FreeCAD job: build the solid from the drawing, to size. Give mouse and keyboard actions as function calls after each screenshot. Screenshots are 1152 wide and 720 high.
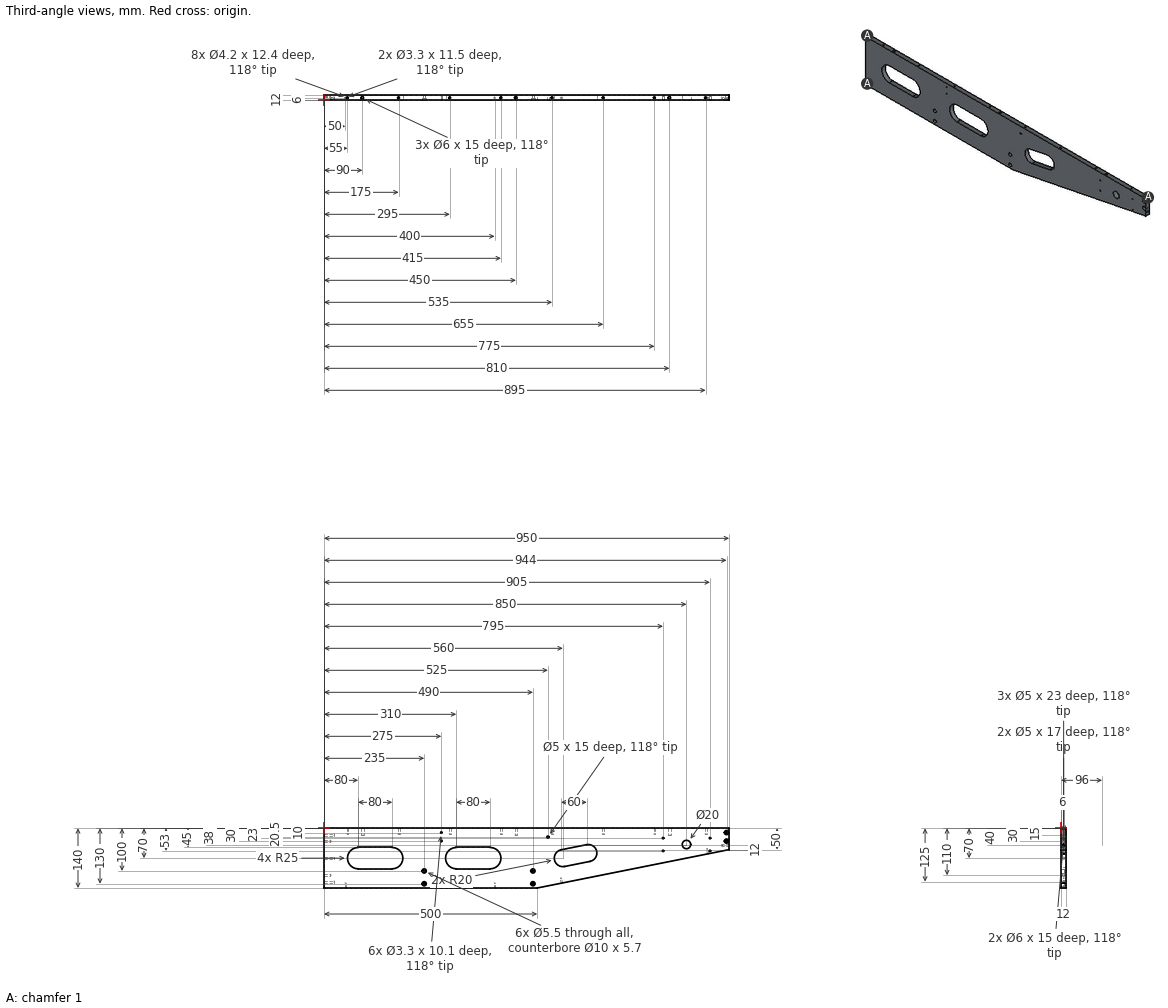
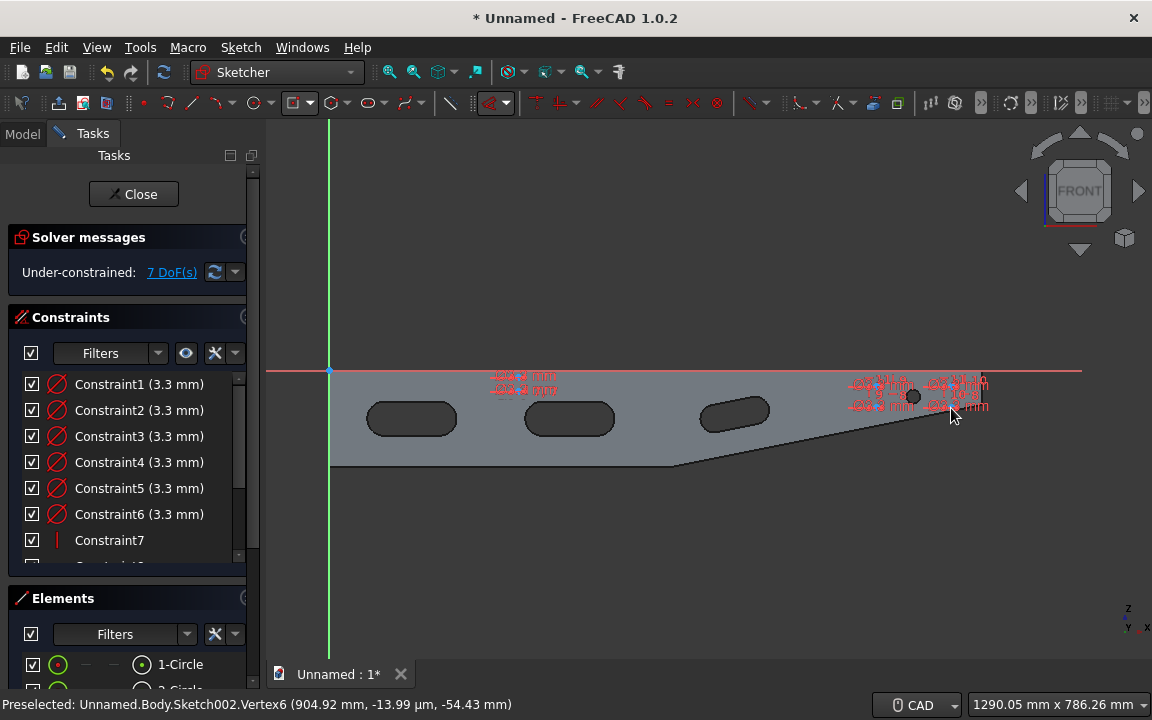
scroll(518, 378, up, 9)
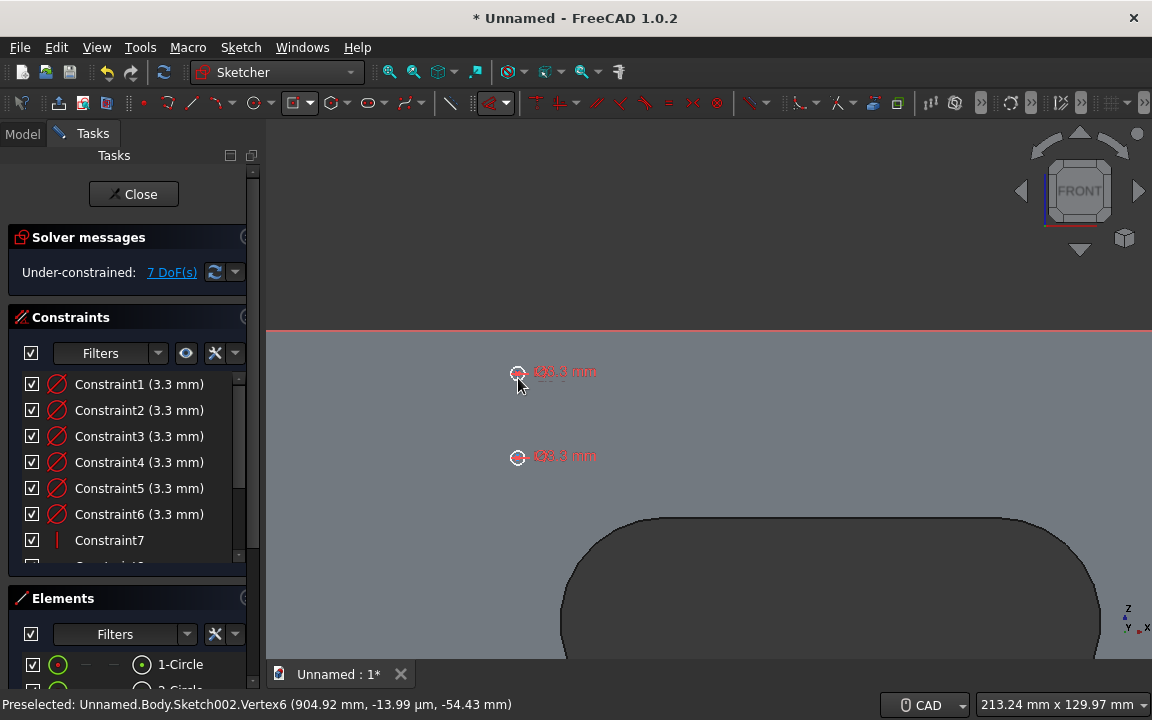
click(518, 374)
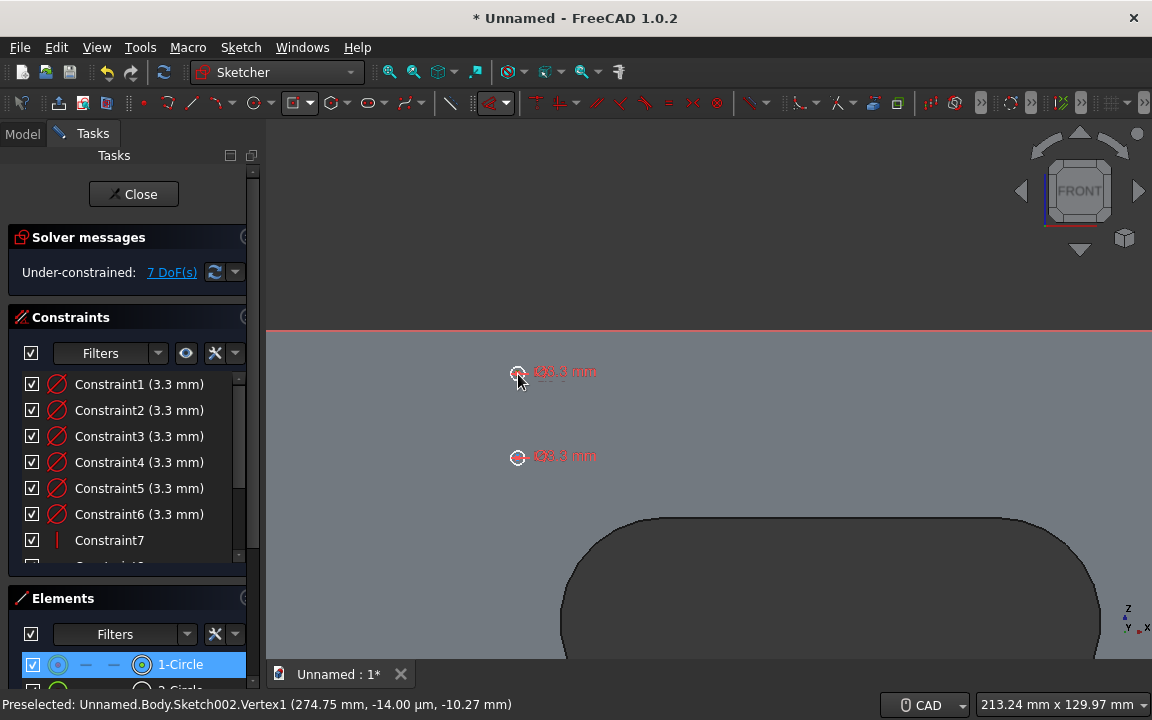
key(i)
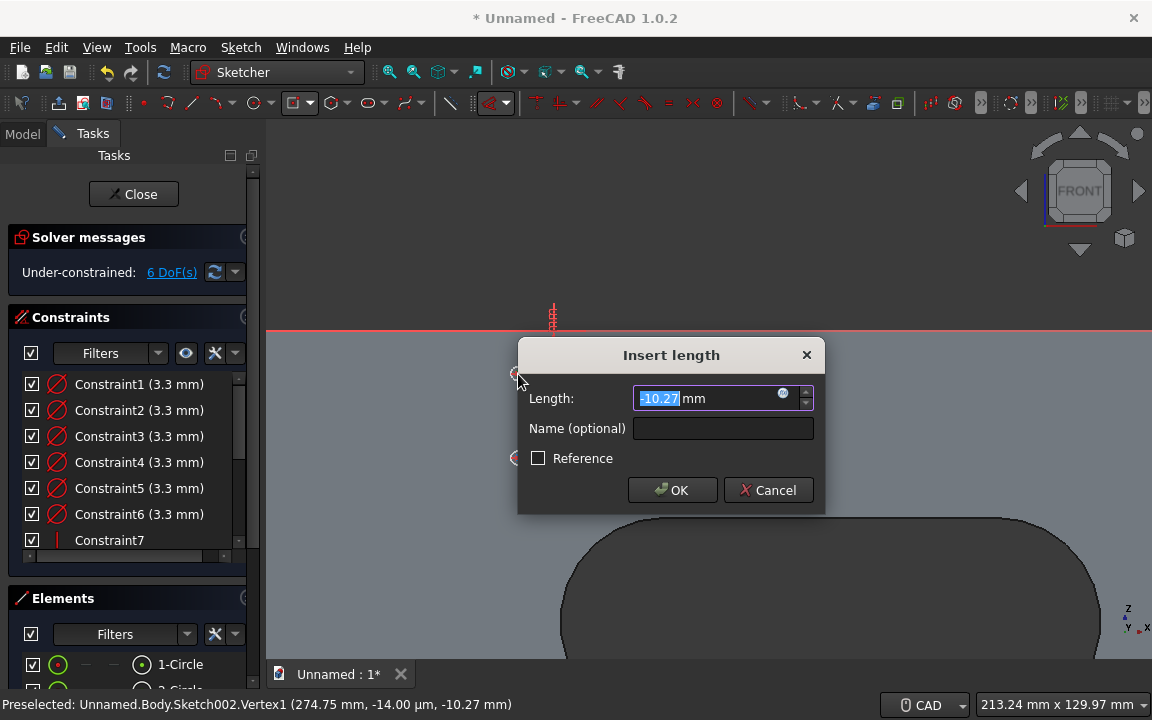
text(-10)
key(Return)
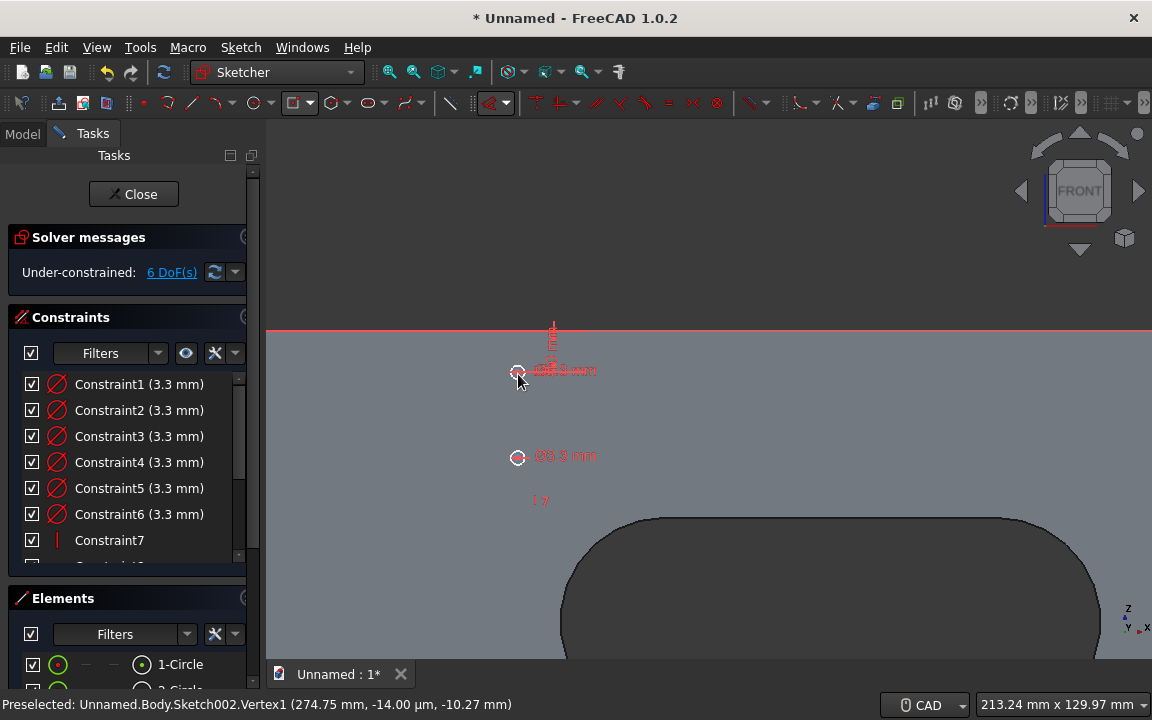
scroll(544, 380, down, 10)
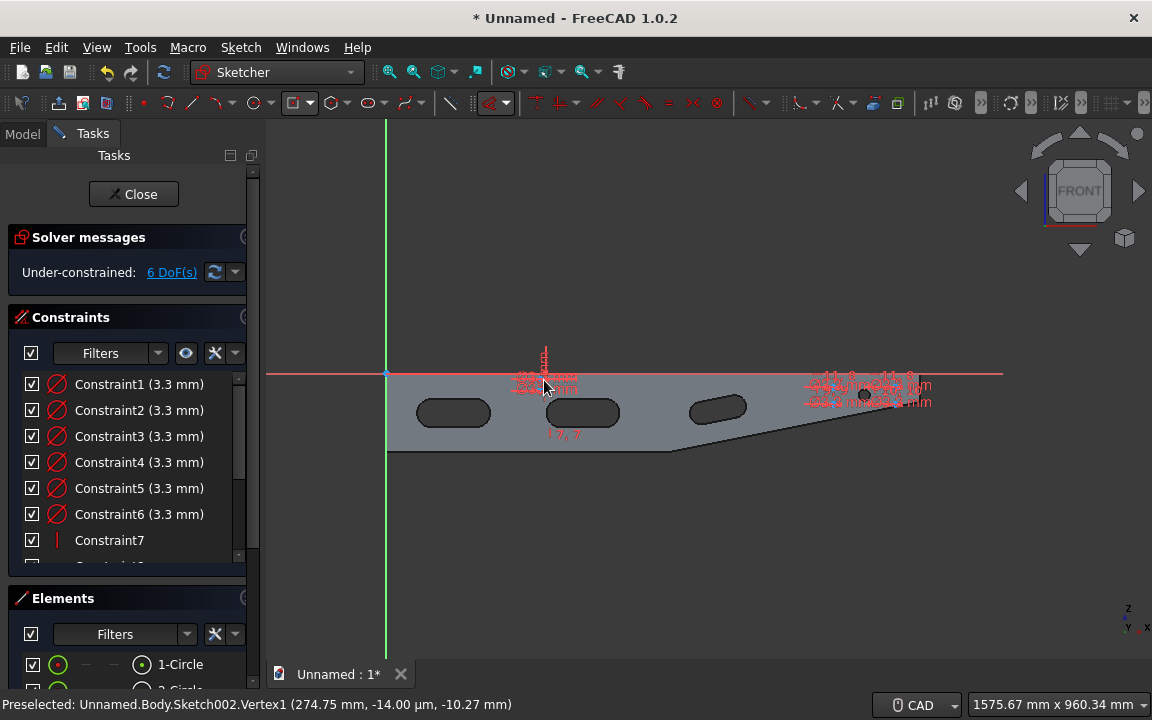
scroll(541, 391, up, 5)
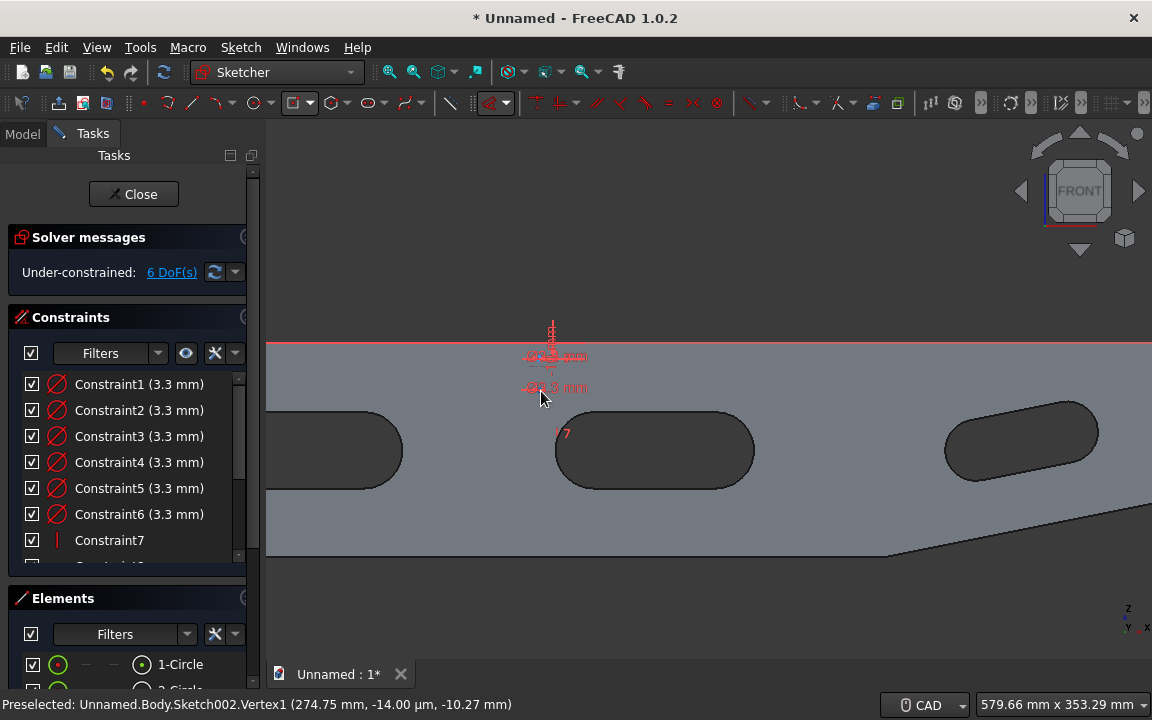
click(540, 390)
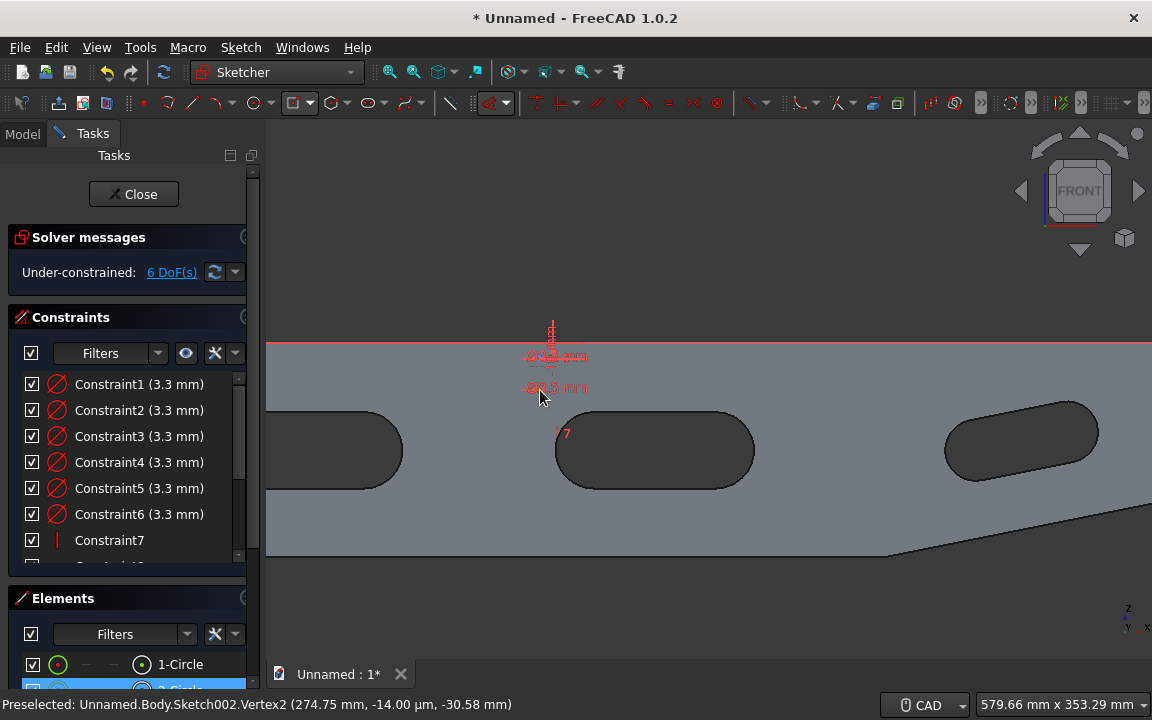
key(i)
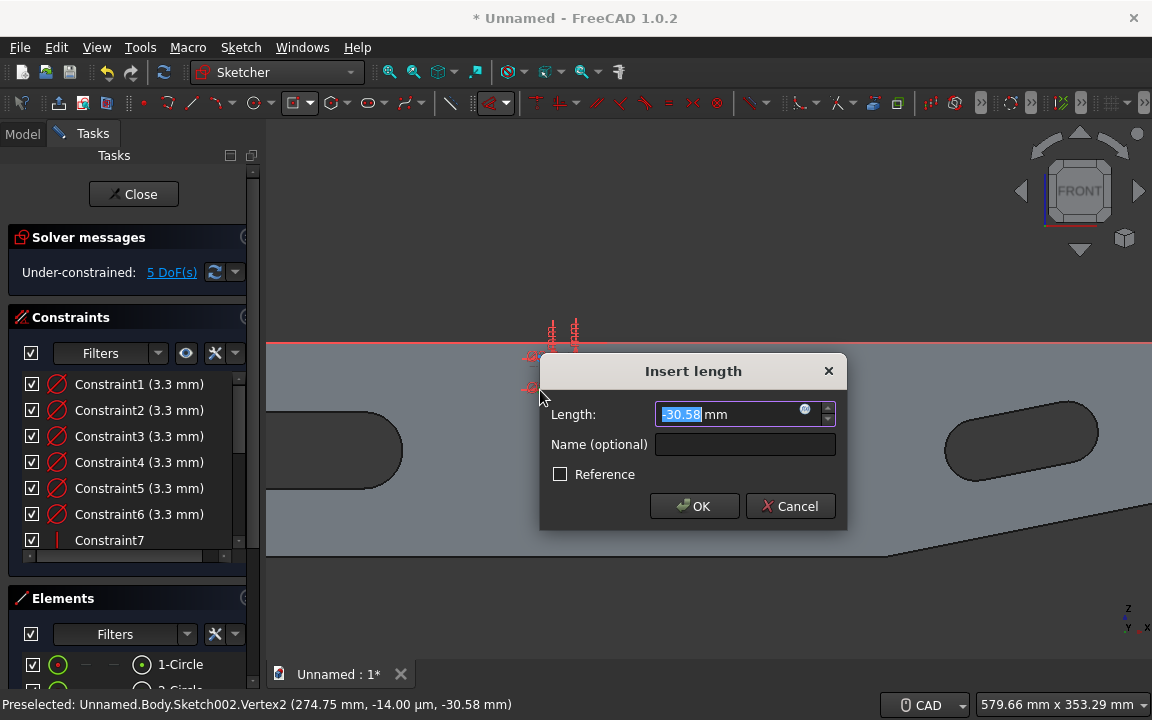
text(-30)
key(Return)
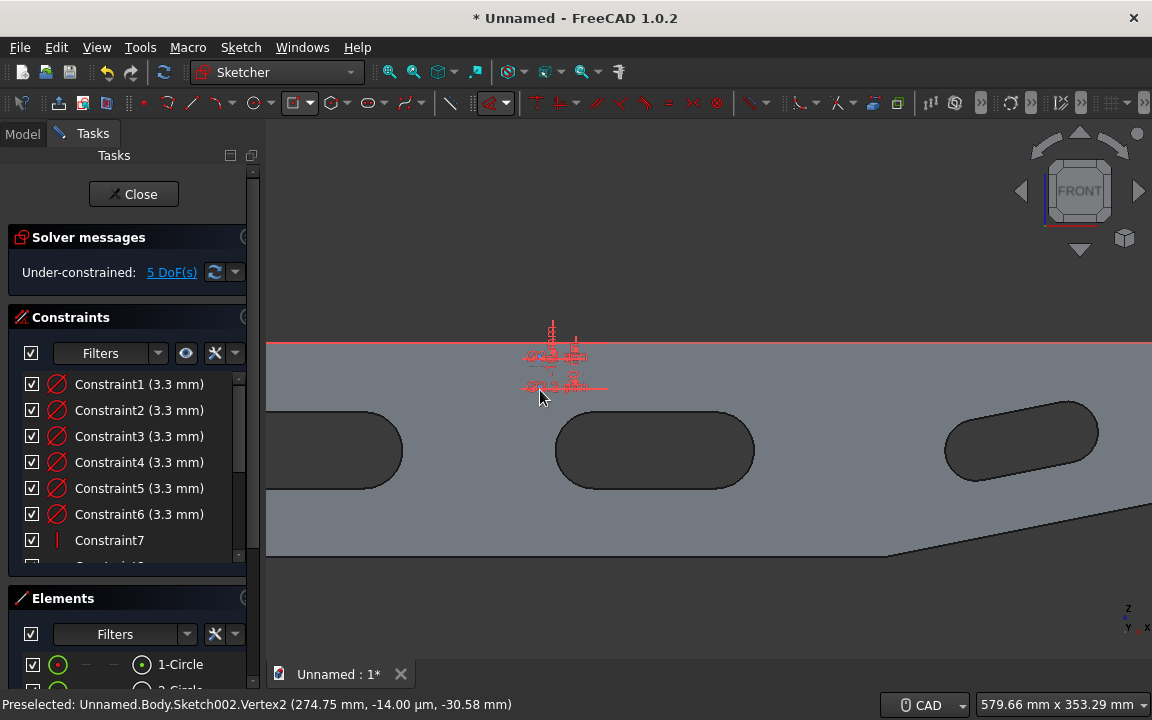
scroll(540, 391, down, 5)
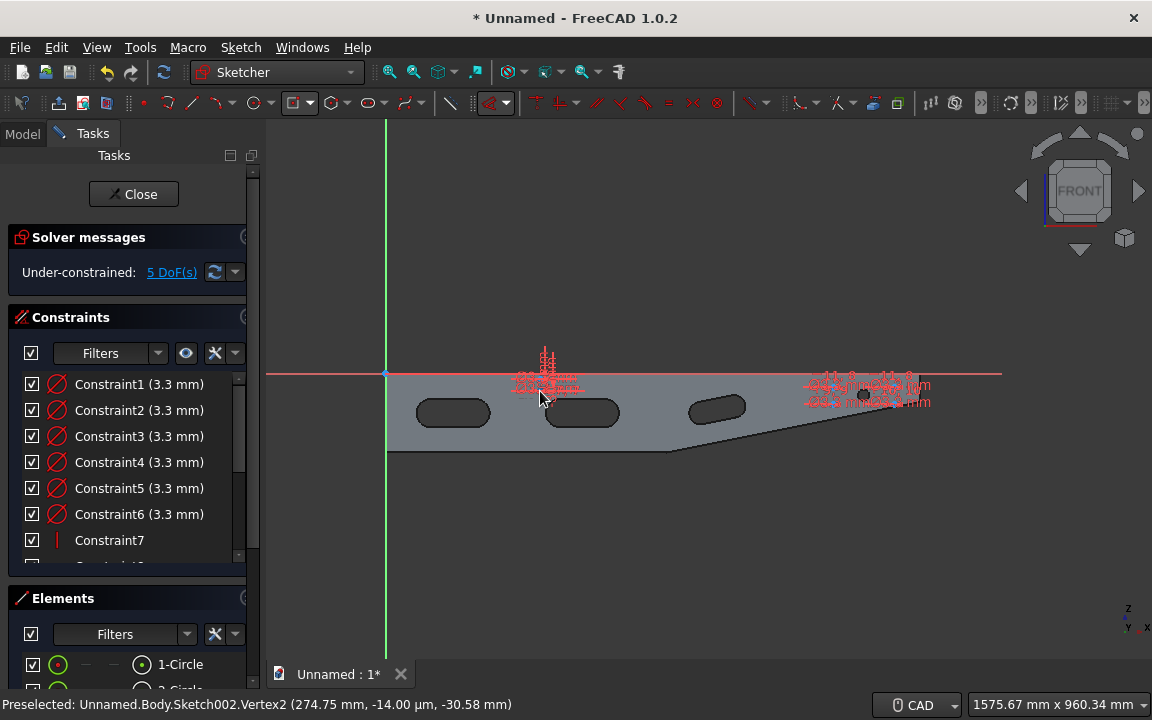
scroll(833, 387, up, 6)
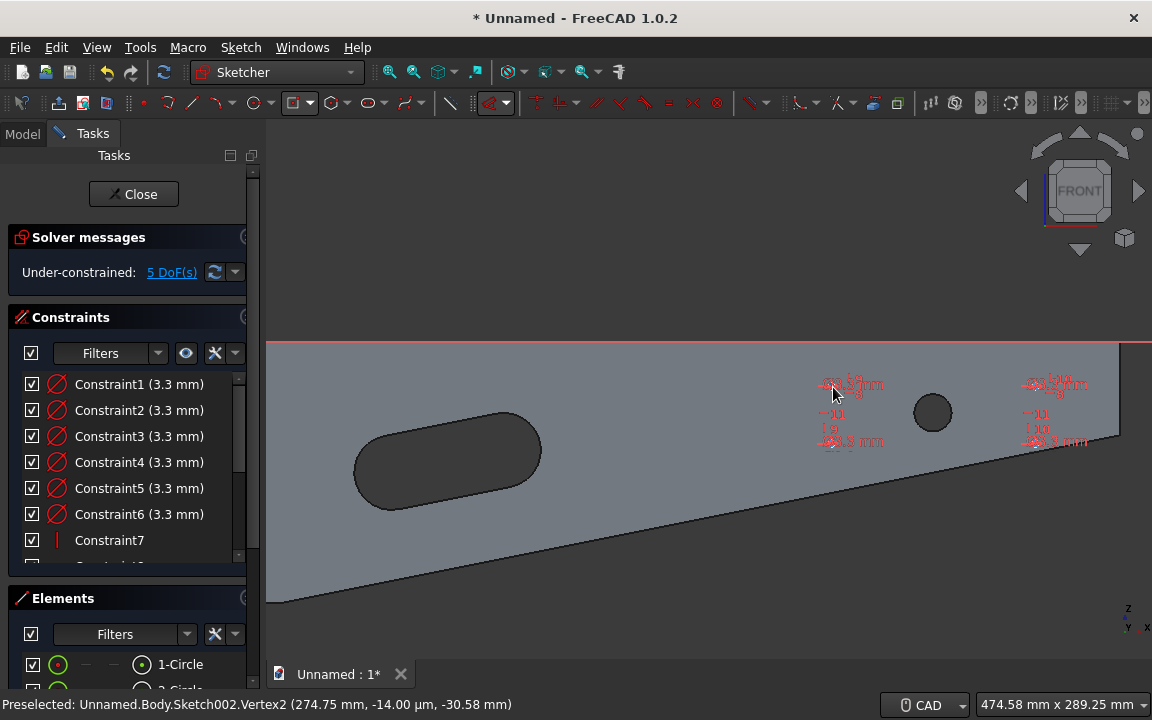
click(832, 386)